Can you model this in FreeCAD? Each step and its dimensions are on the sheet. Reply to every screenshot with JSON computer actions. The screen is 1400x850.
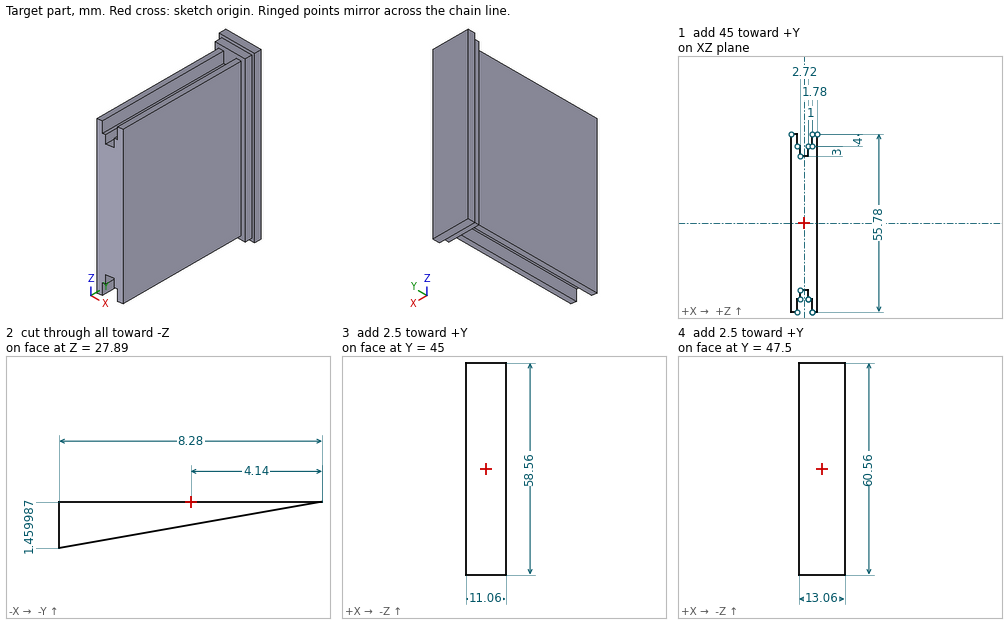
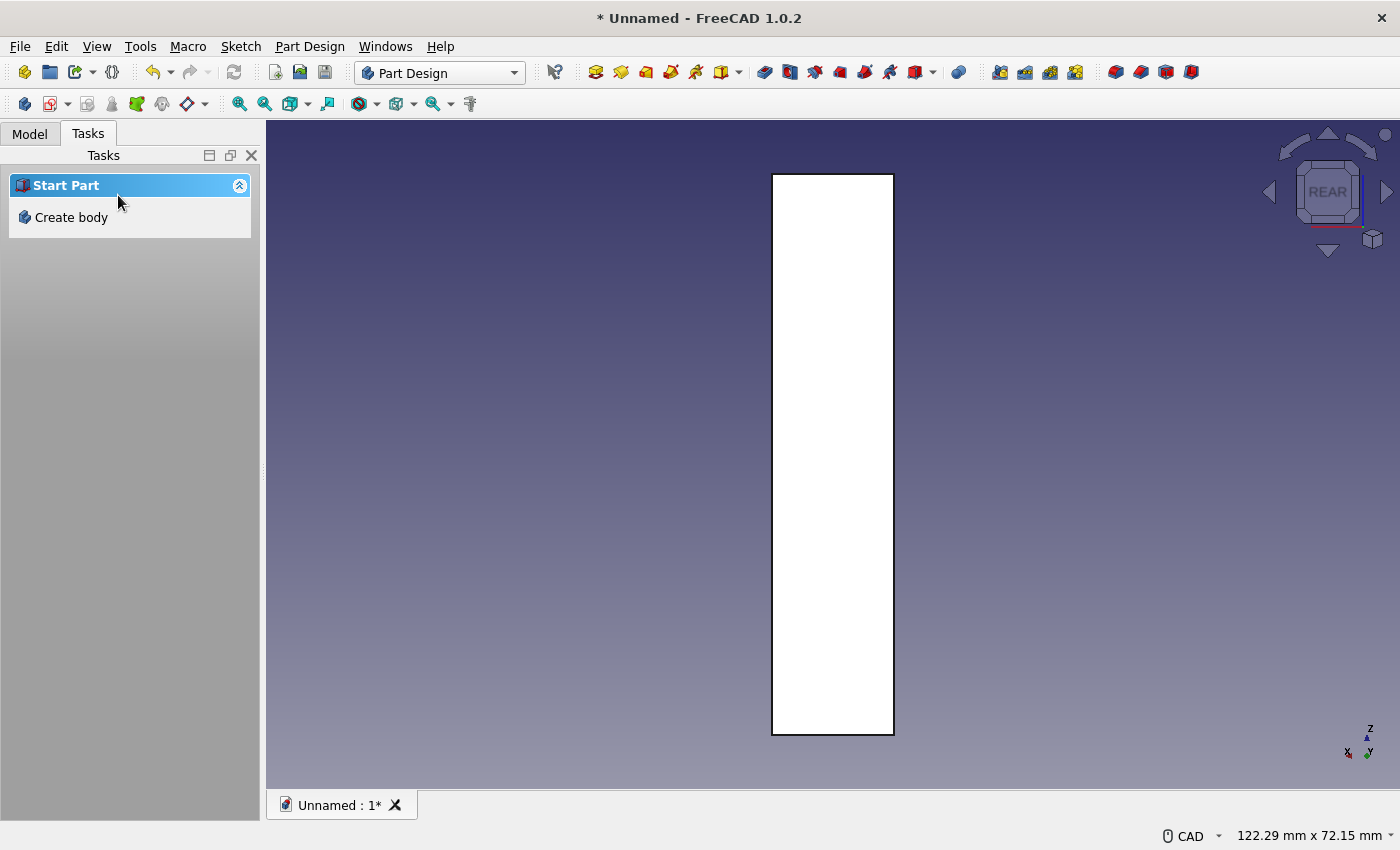
{"action": "key", "text": "0"}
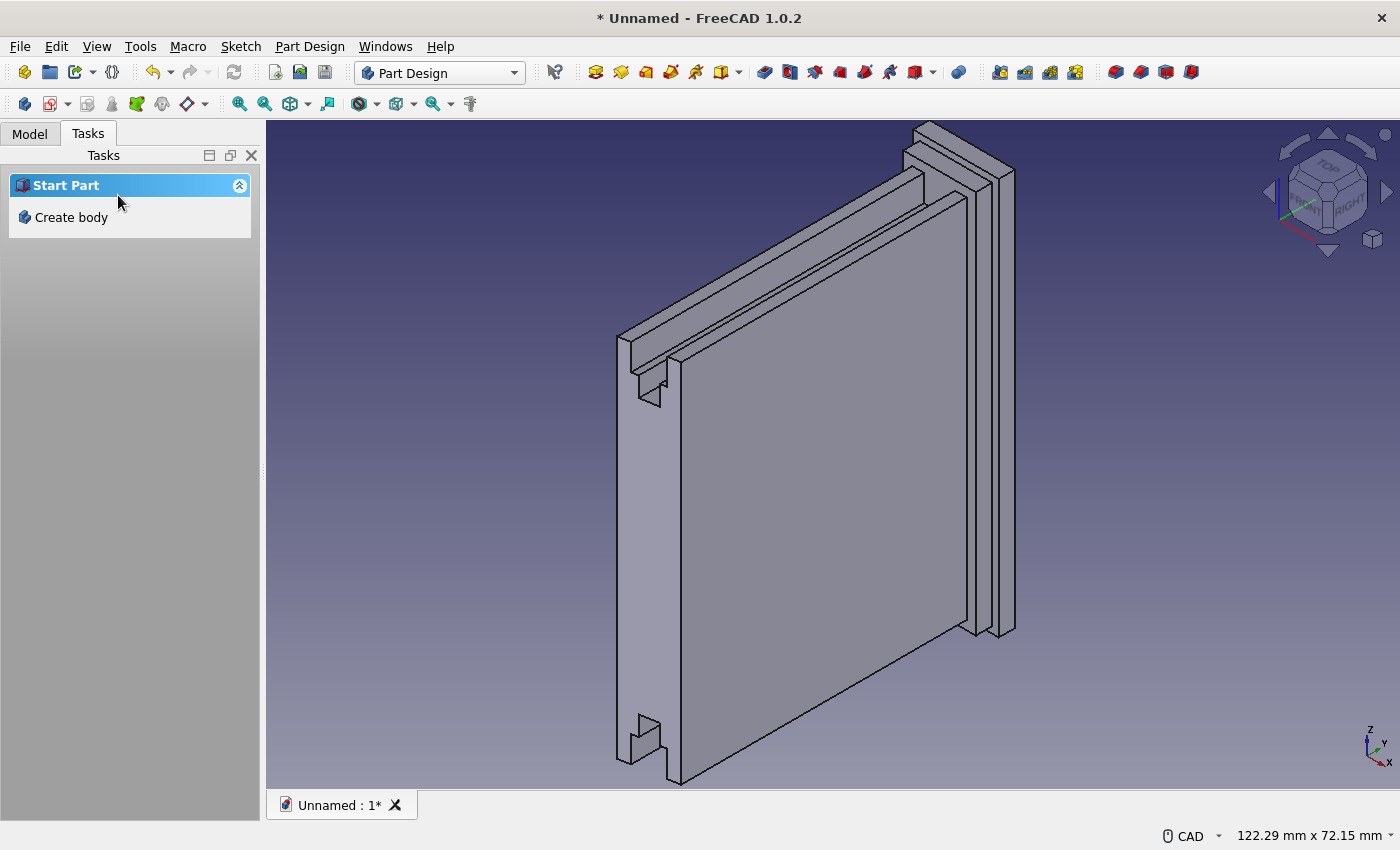
{"action": "left_click", "coordinate": [240, 104]}